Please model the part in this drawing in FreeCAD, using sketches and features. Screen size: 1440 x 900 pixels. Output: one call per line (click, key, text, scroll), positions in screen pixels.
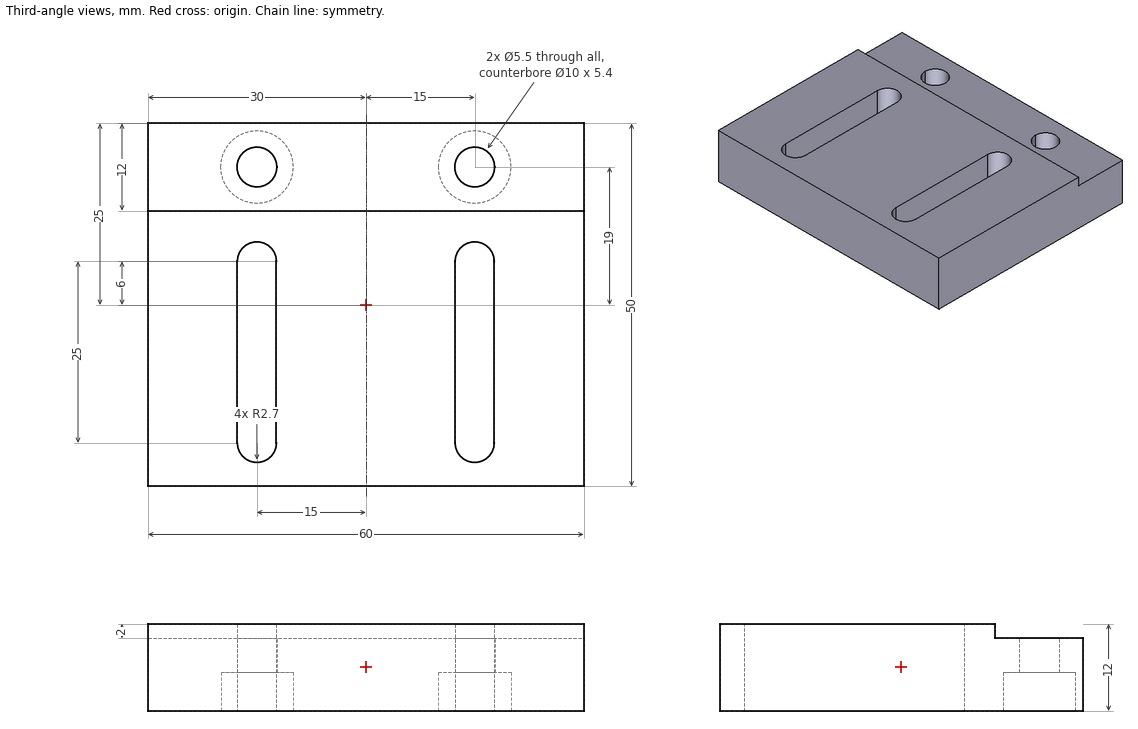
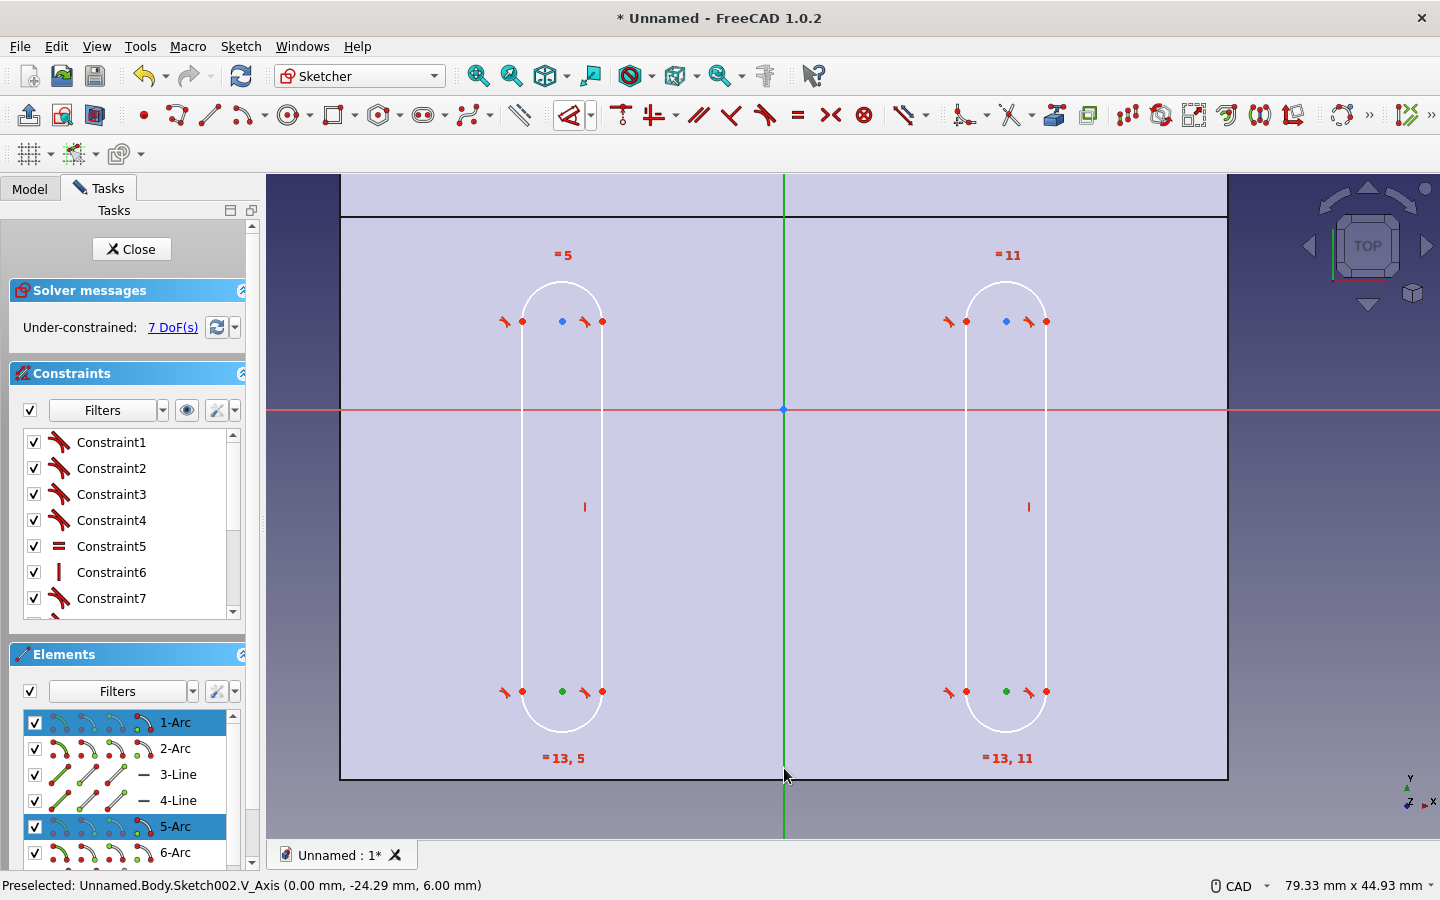
key(s)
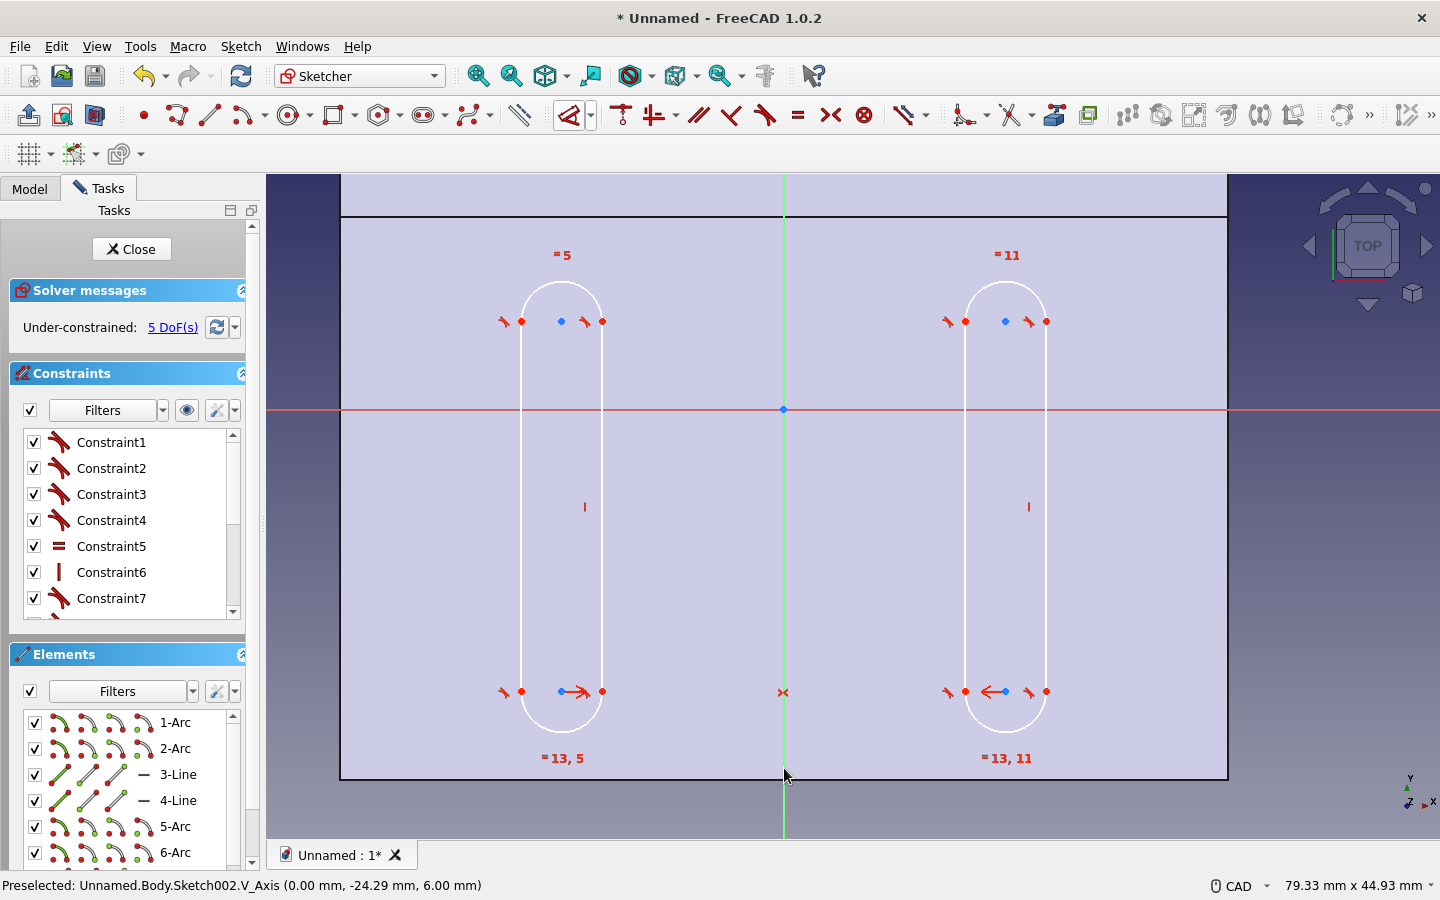
click(538, 725)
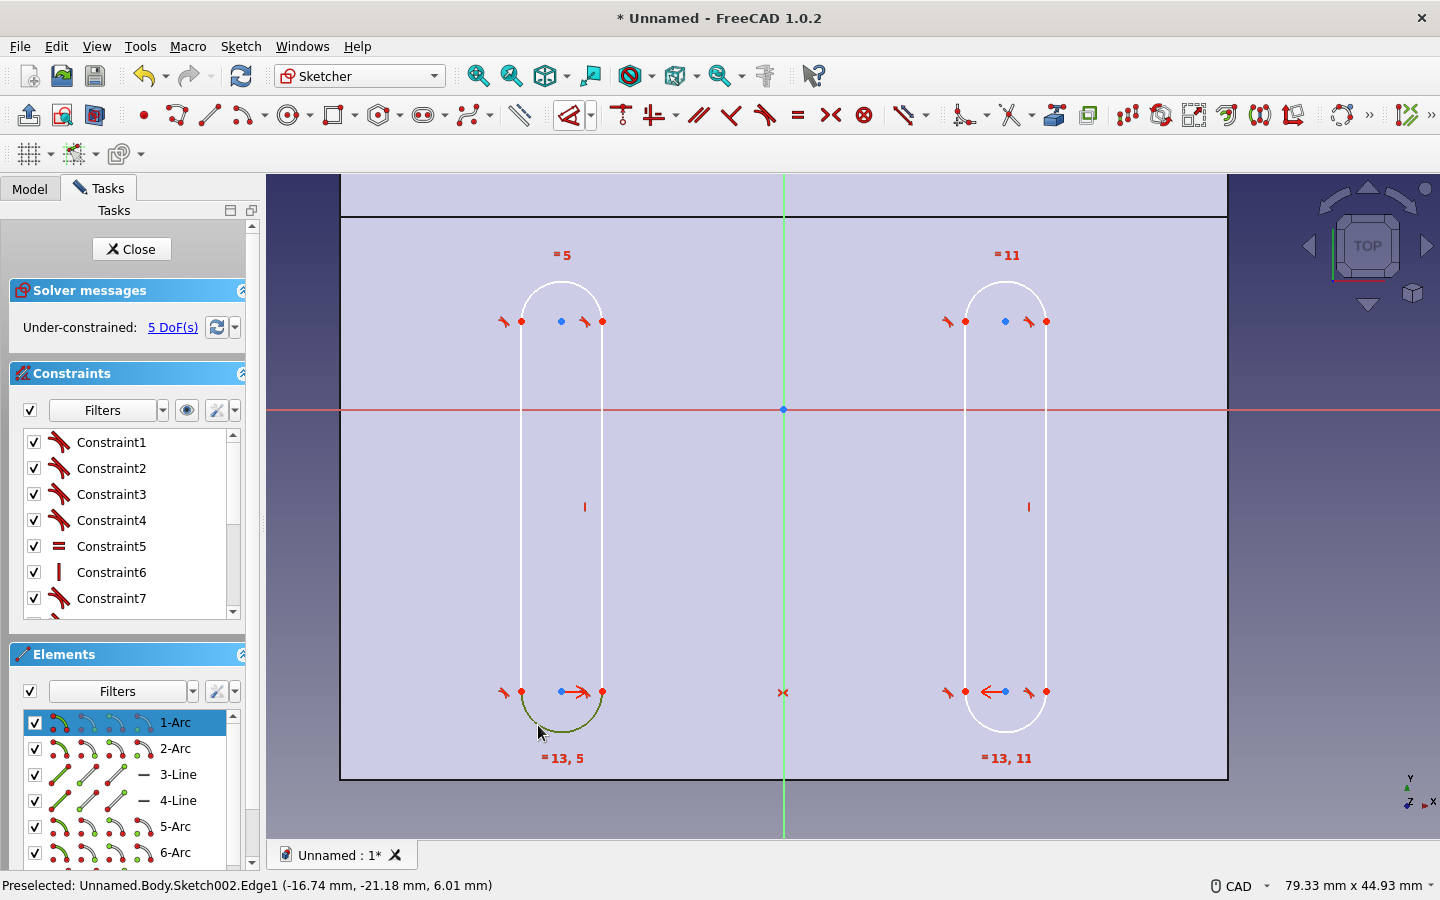
click(590, 116)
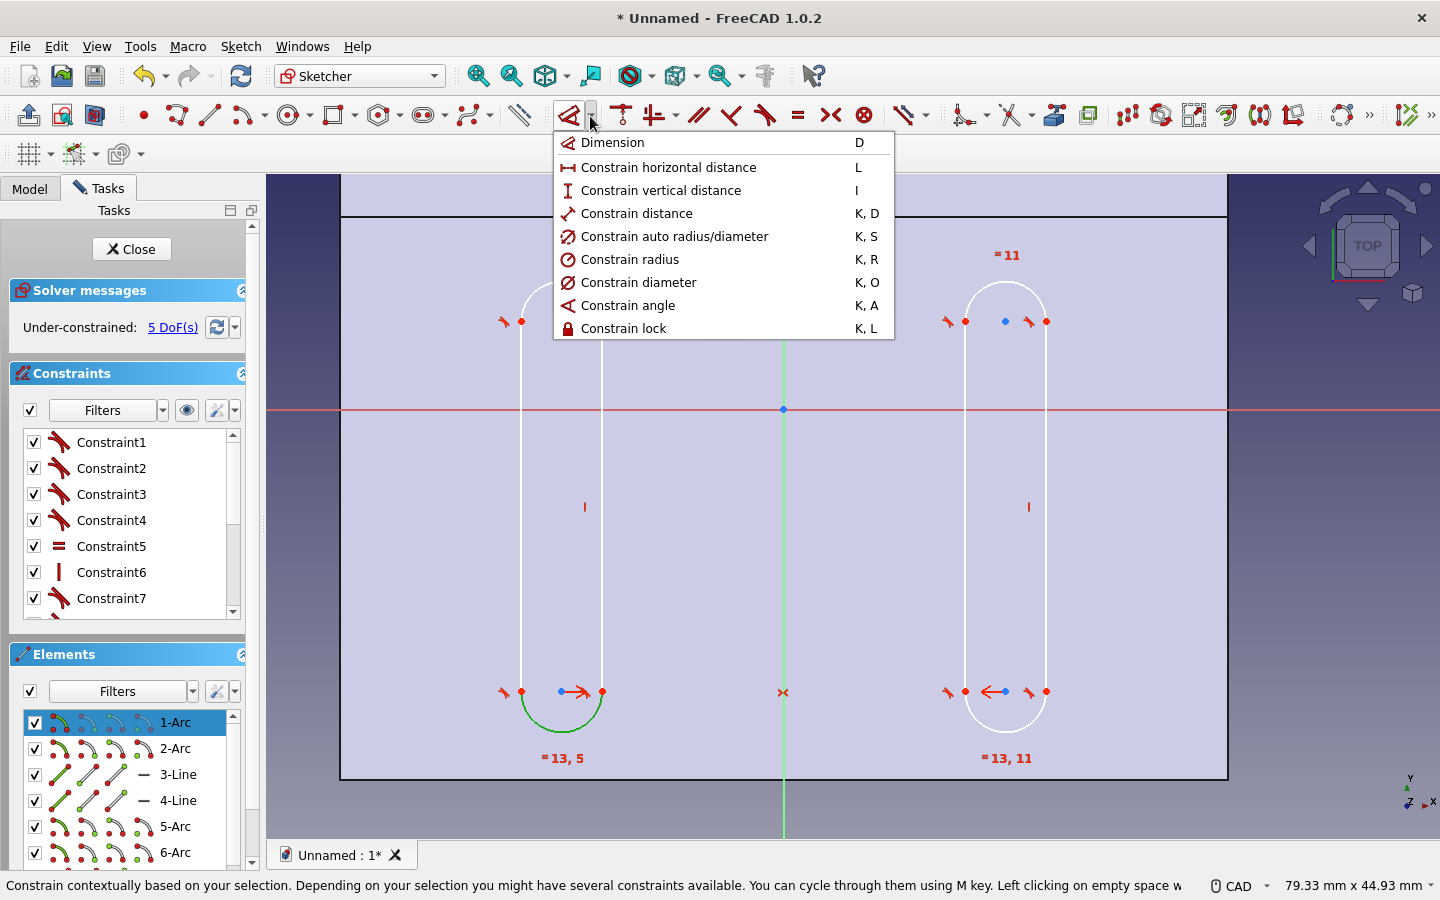
click(724, 260)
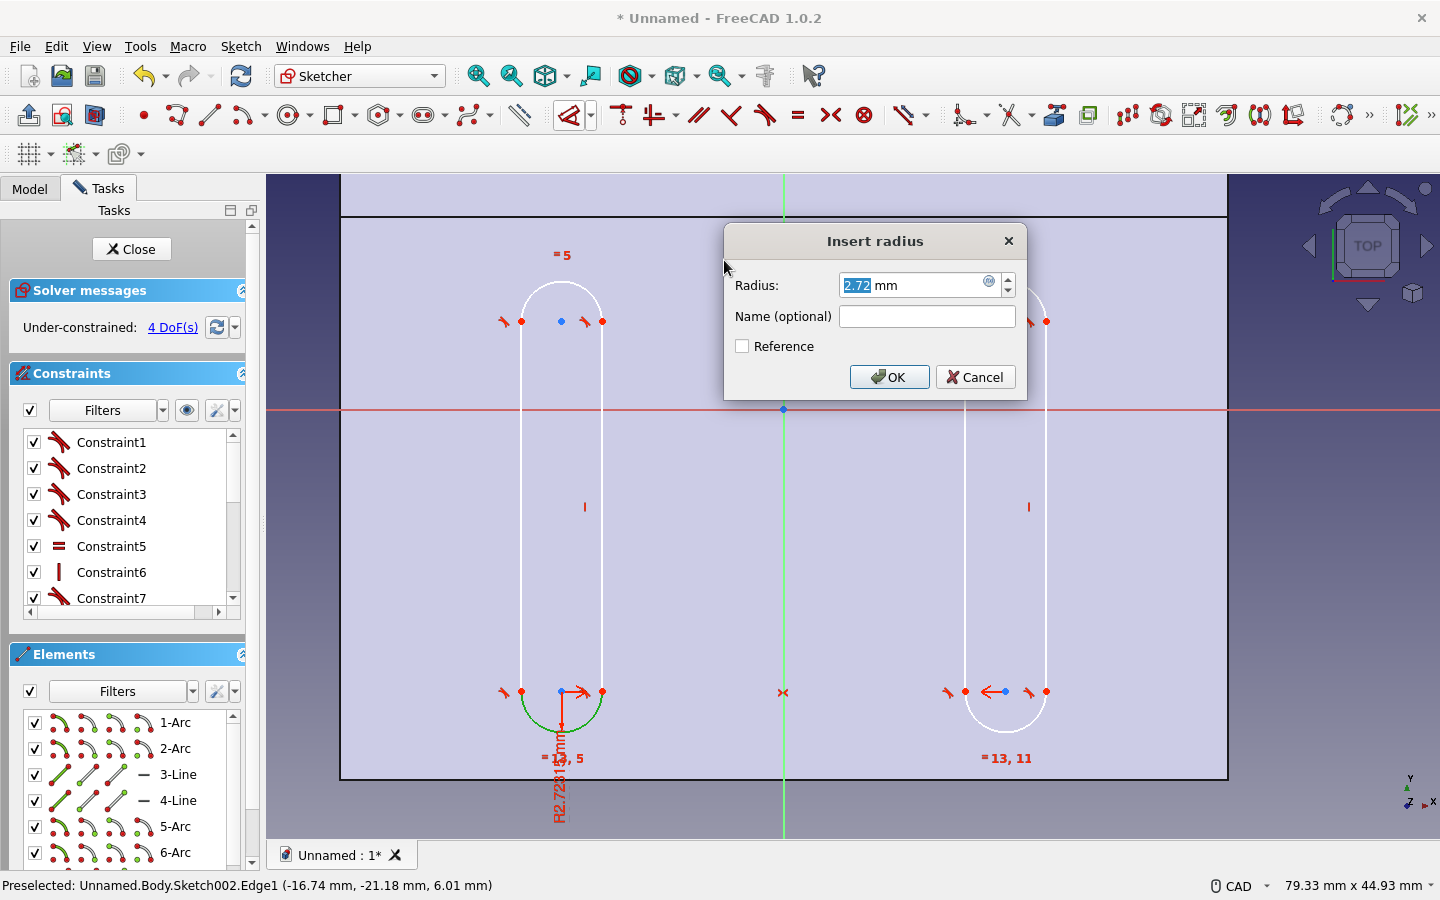
text(2.7)
key(Return)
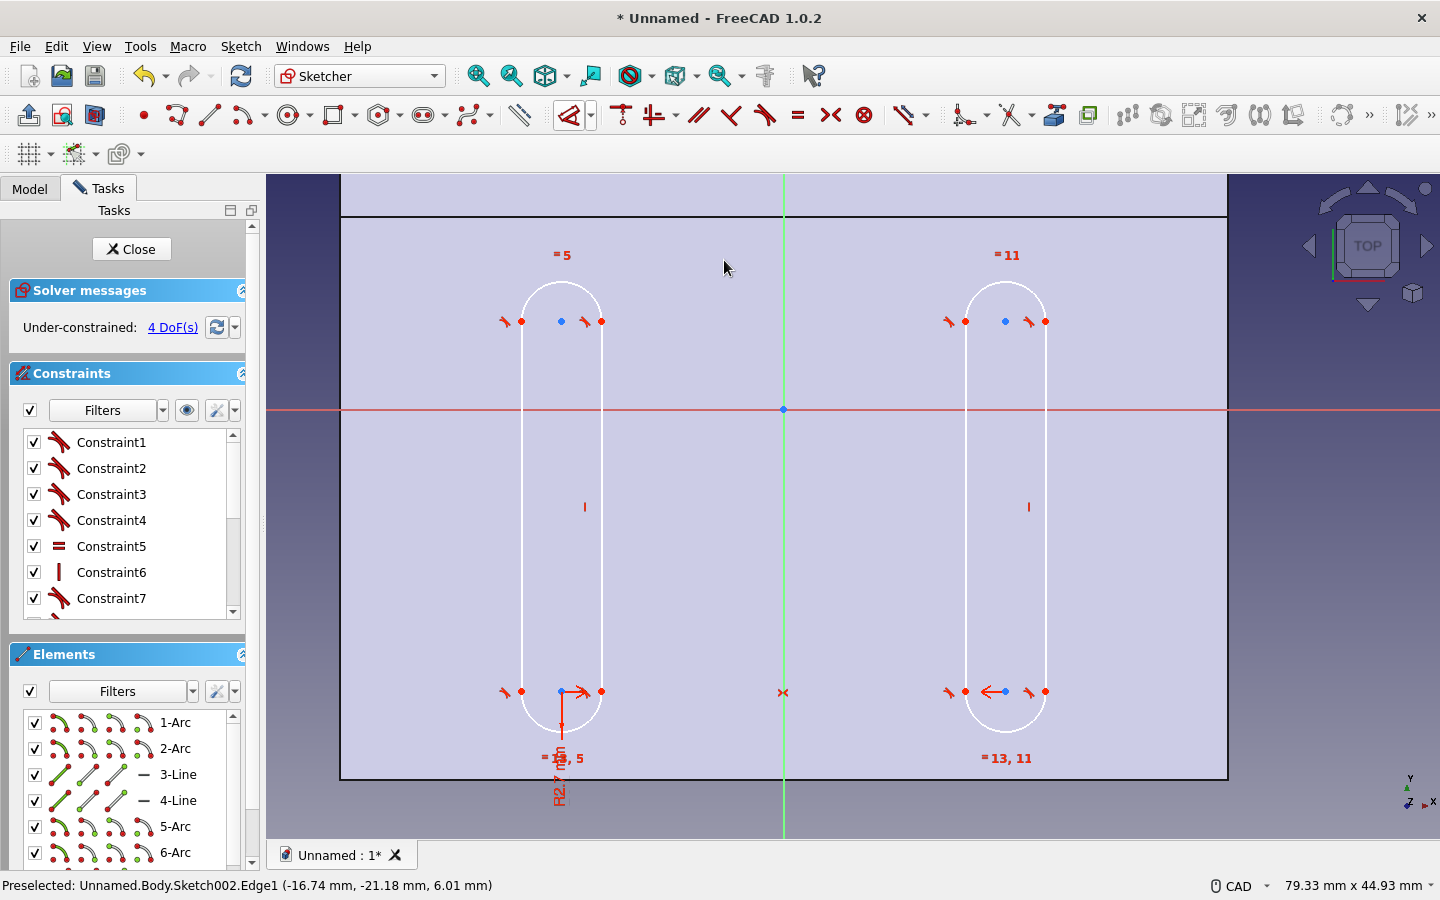
click(522, 581)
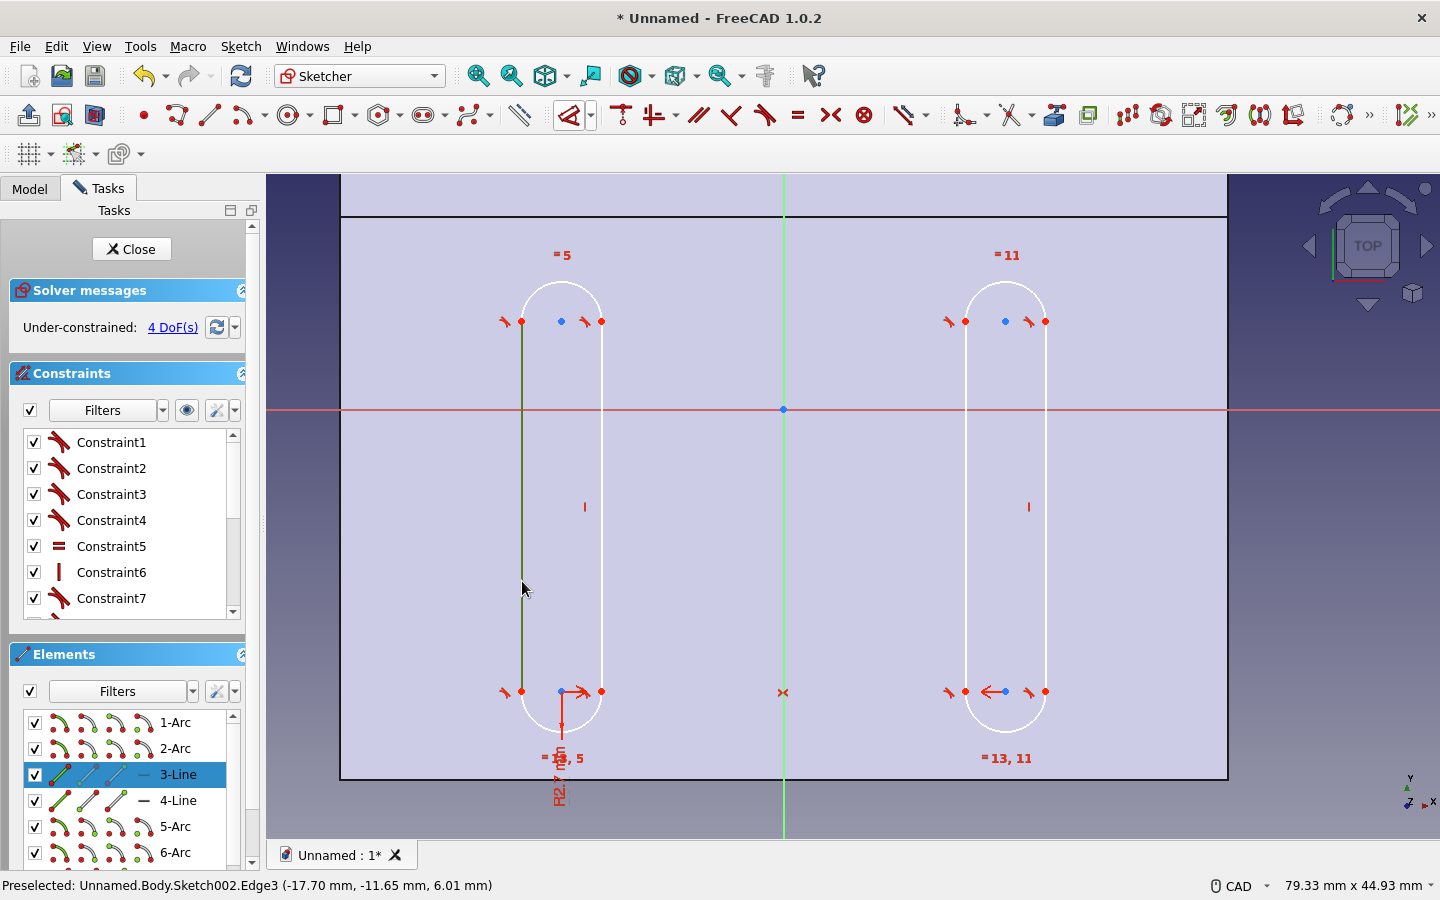
click(590, 116)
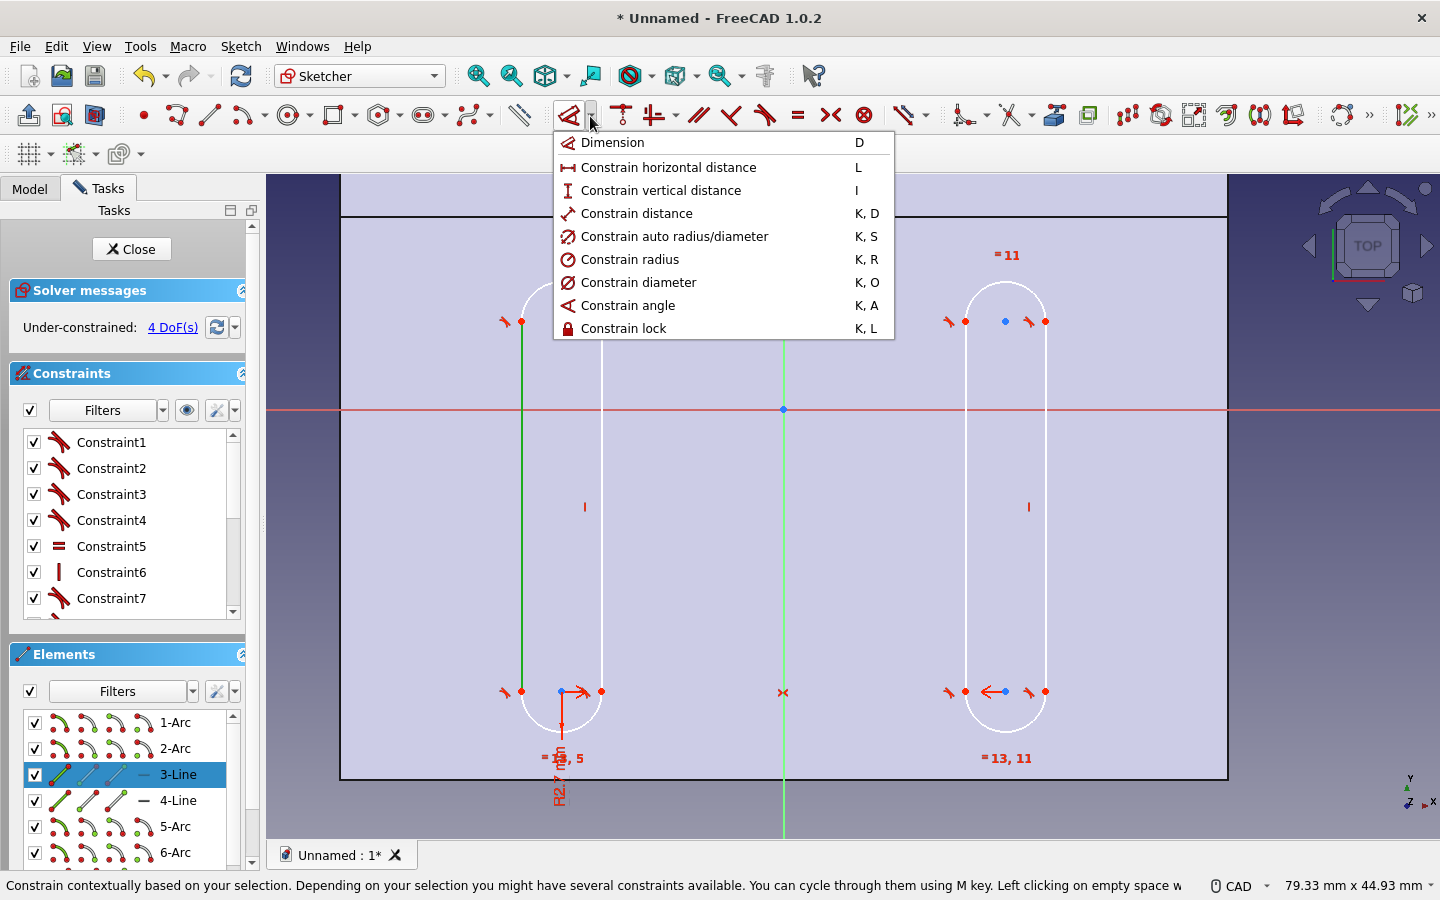
click(724, 190)